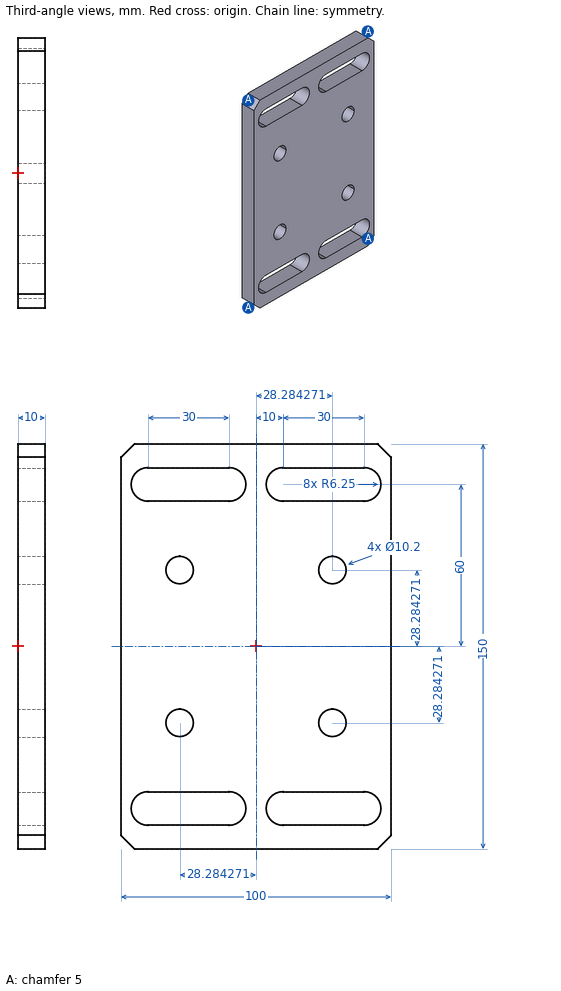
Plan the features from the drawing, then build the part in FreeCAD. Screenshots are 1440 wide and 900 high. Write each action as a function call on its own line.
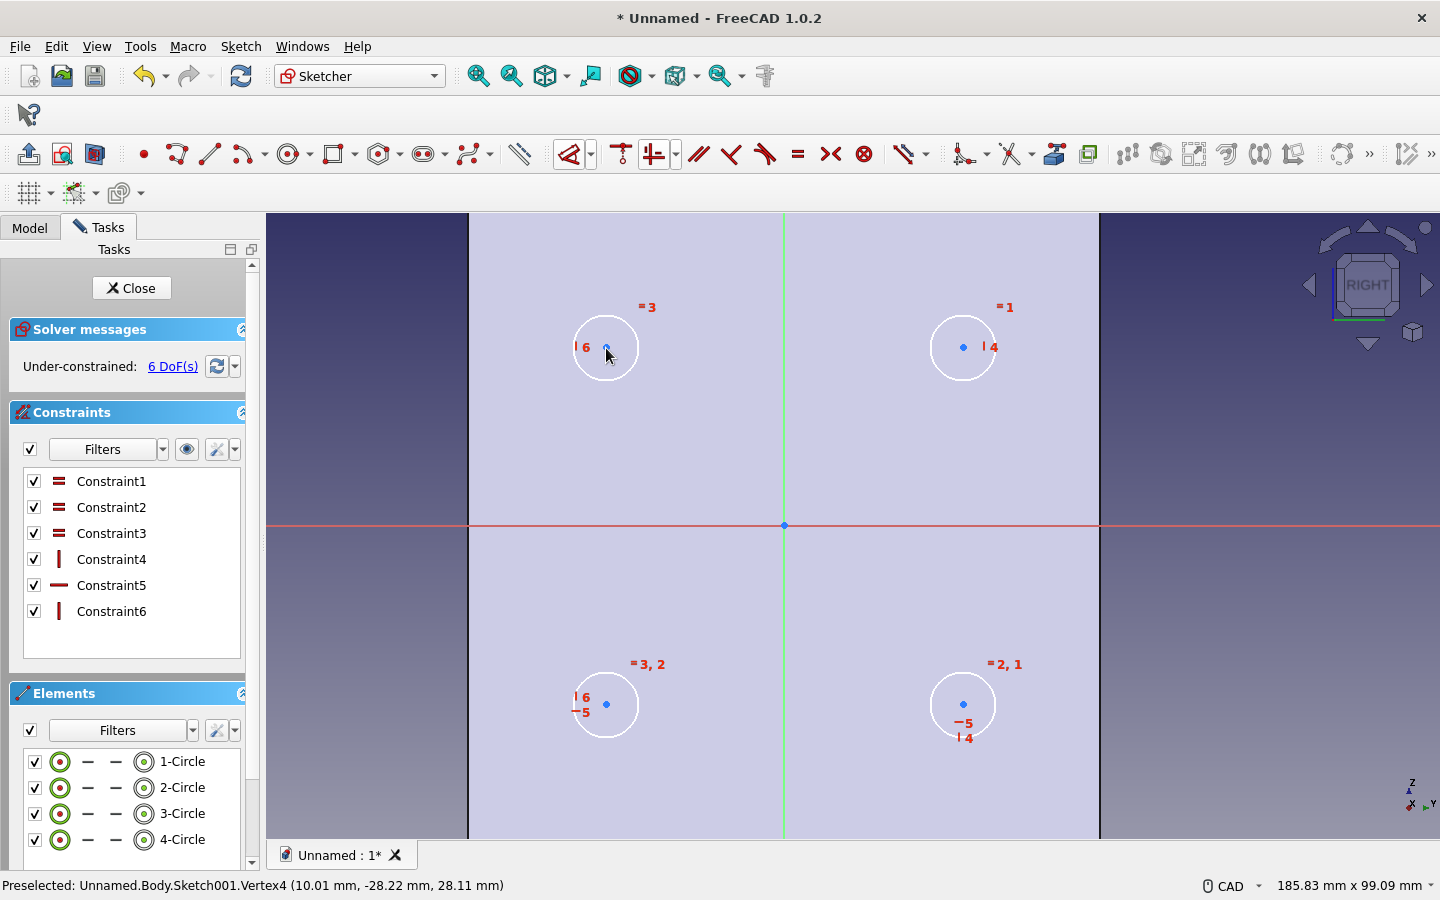
click(963, 348)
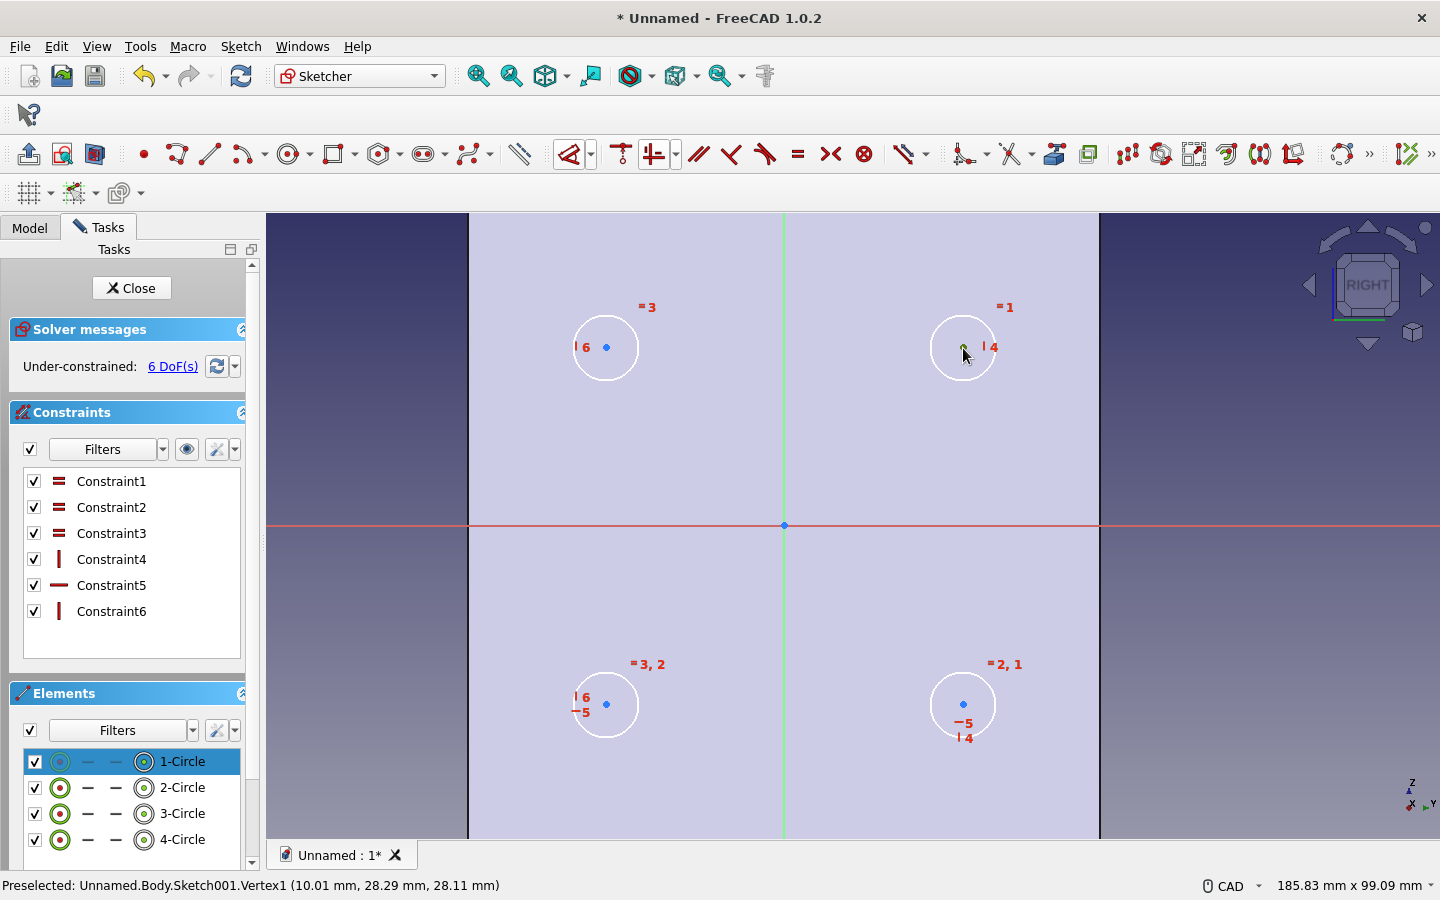
click(606, 348)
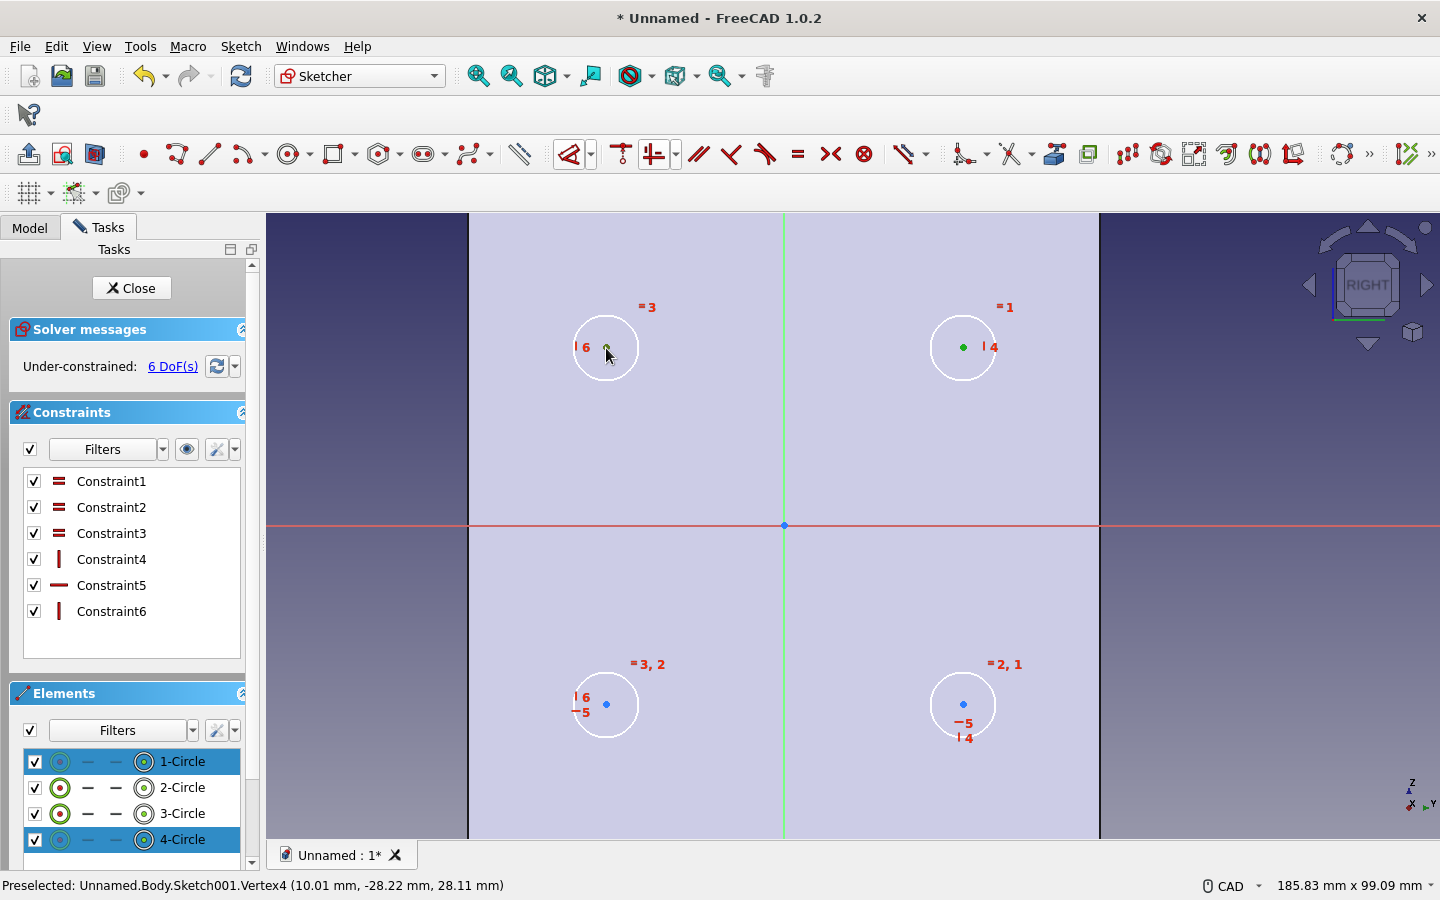
click(676, 154)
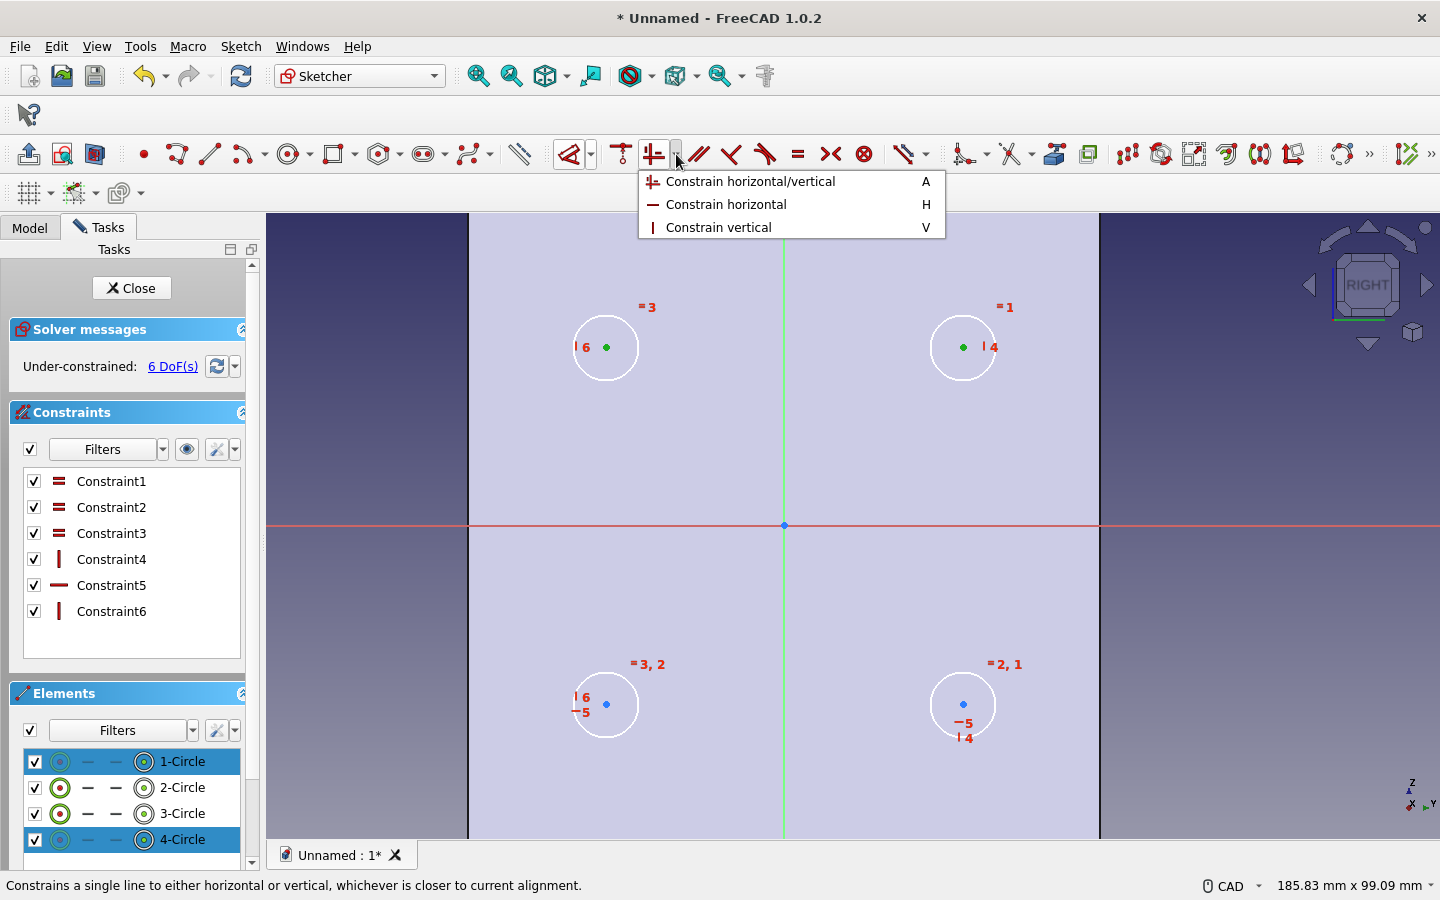
click(792, 204)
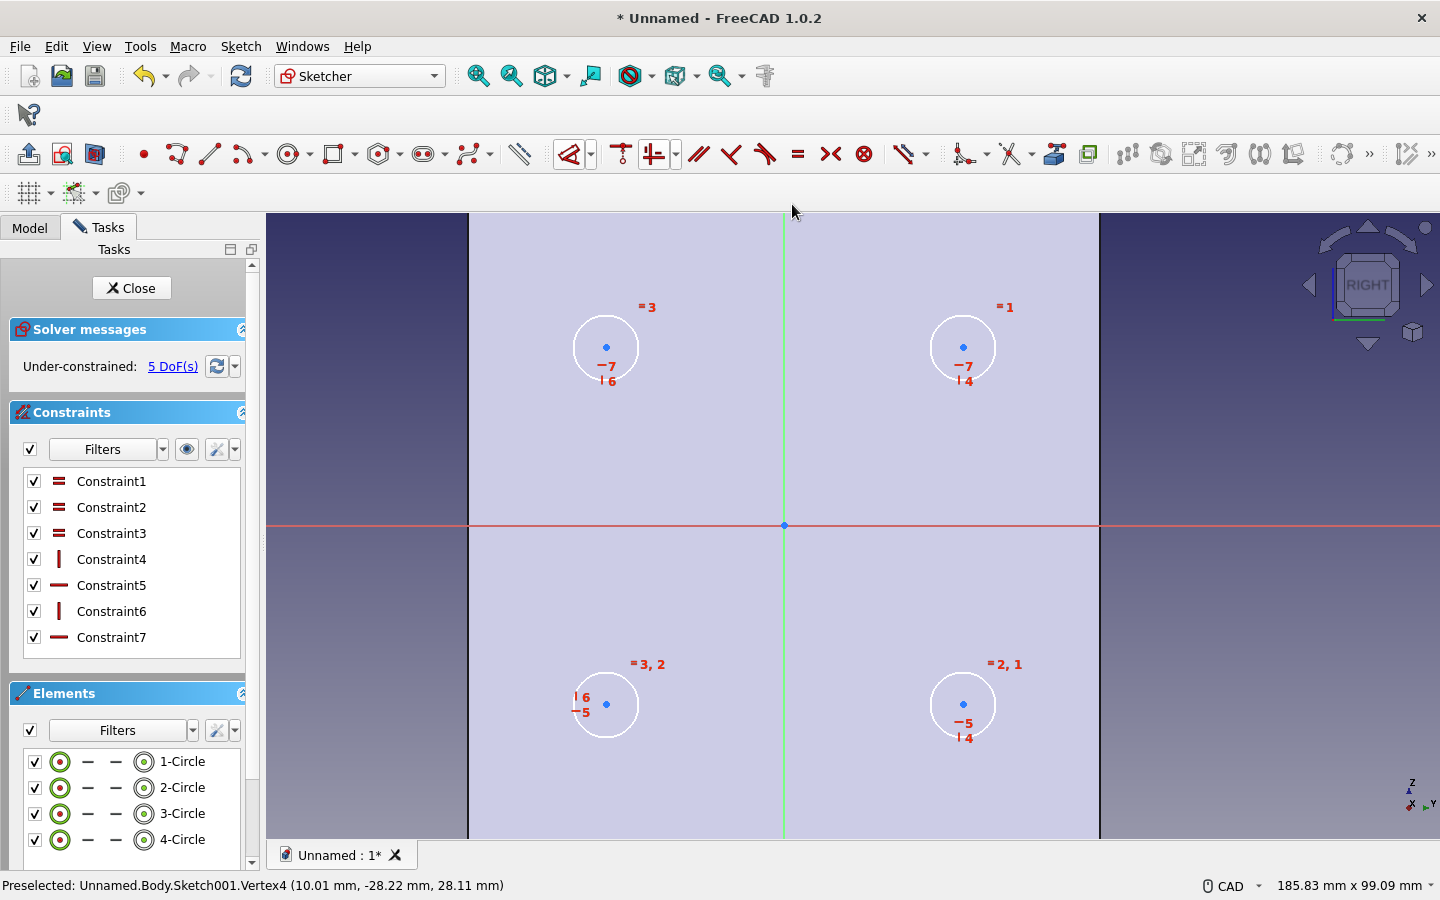
click(568, 154)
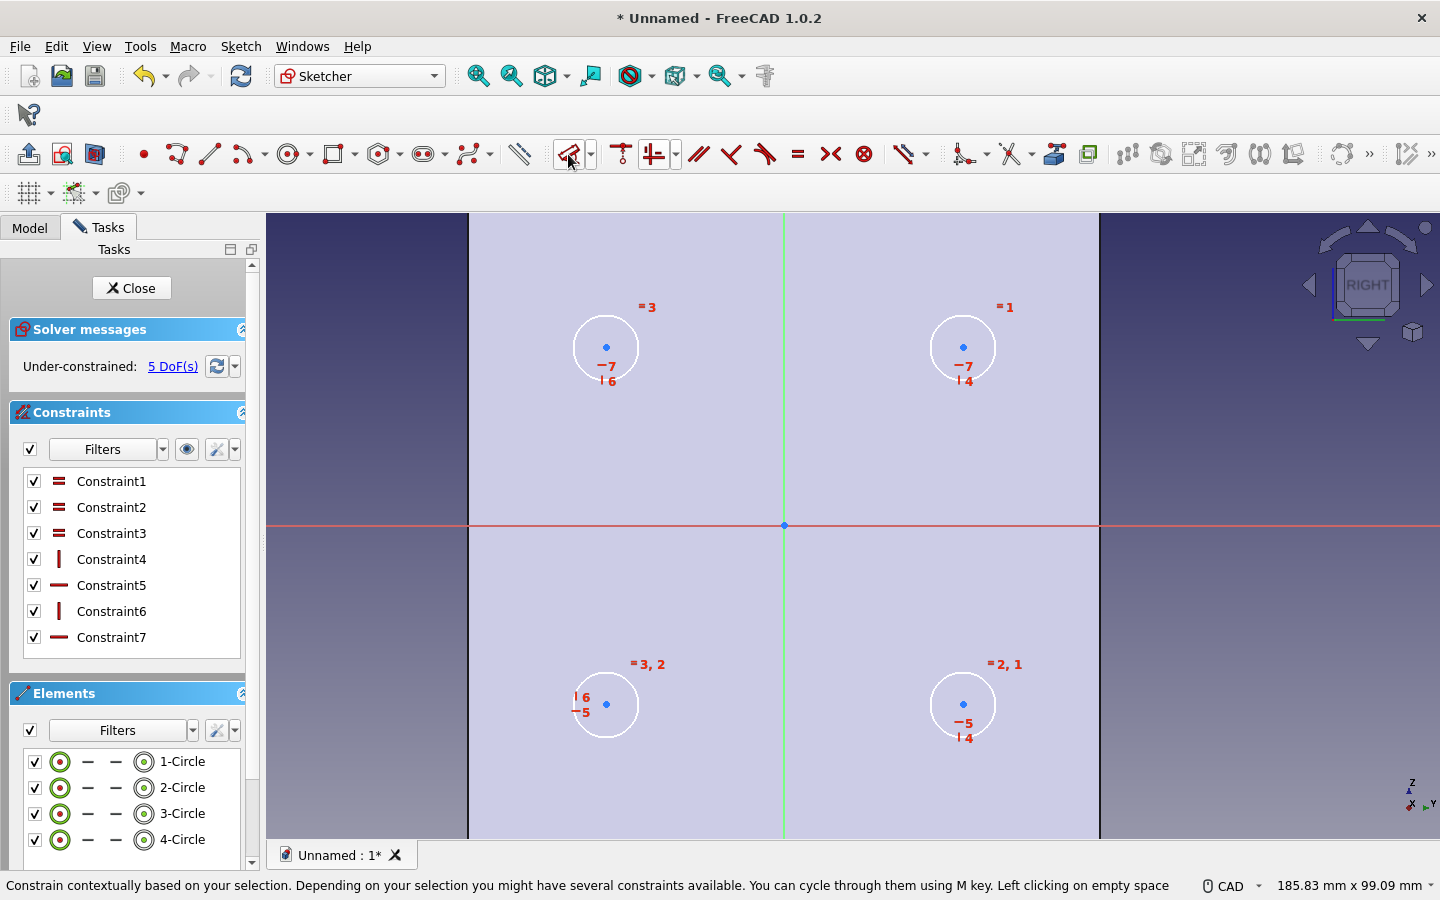
click(986, 325)
click(1009, 302)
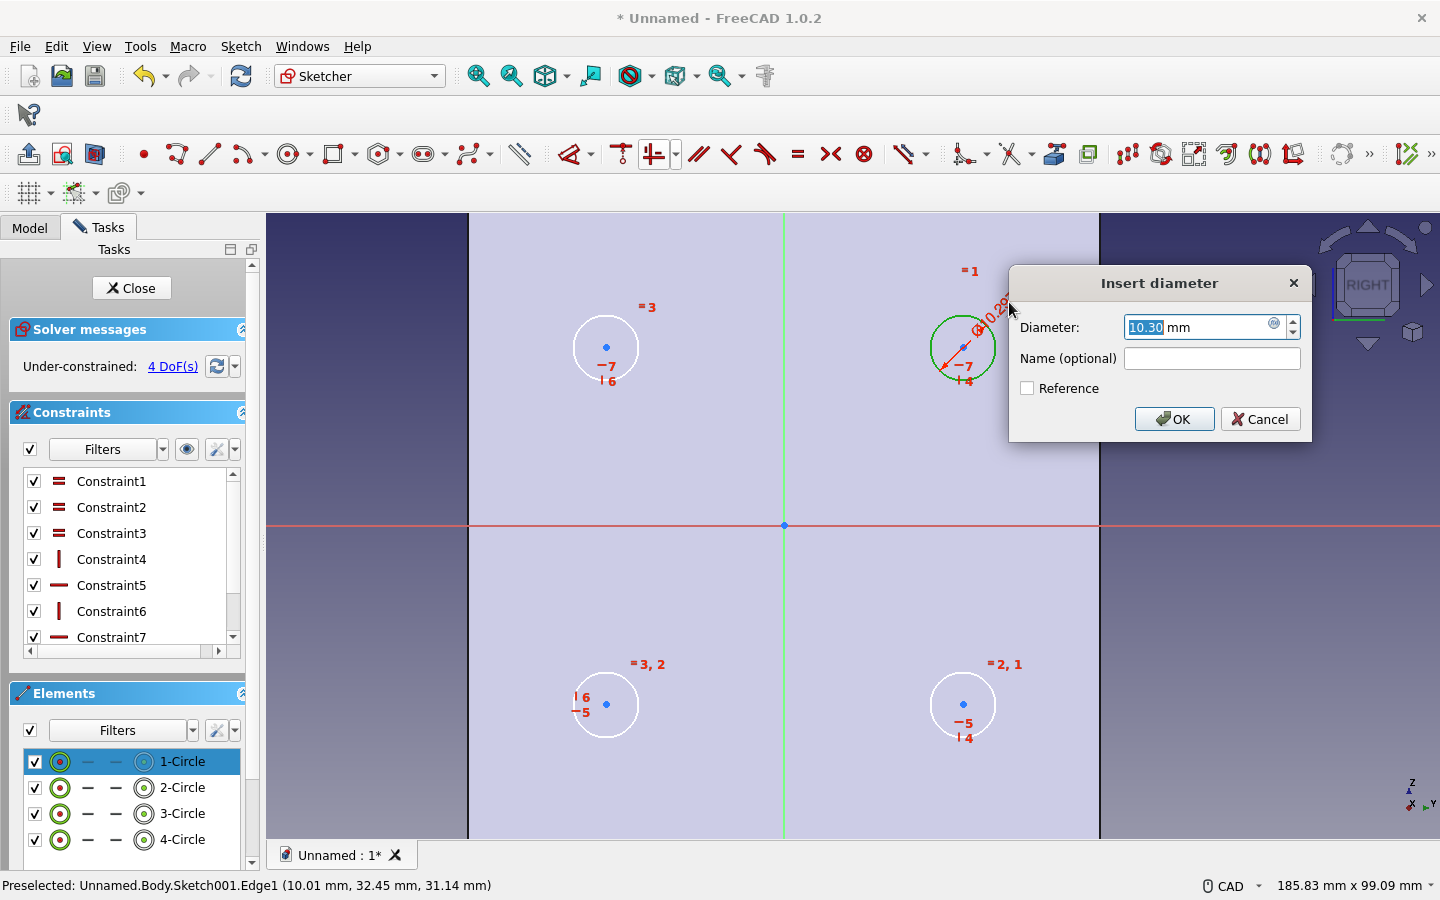
text(10.2)
key(Return)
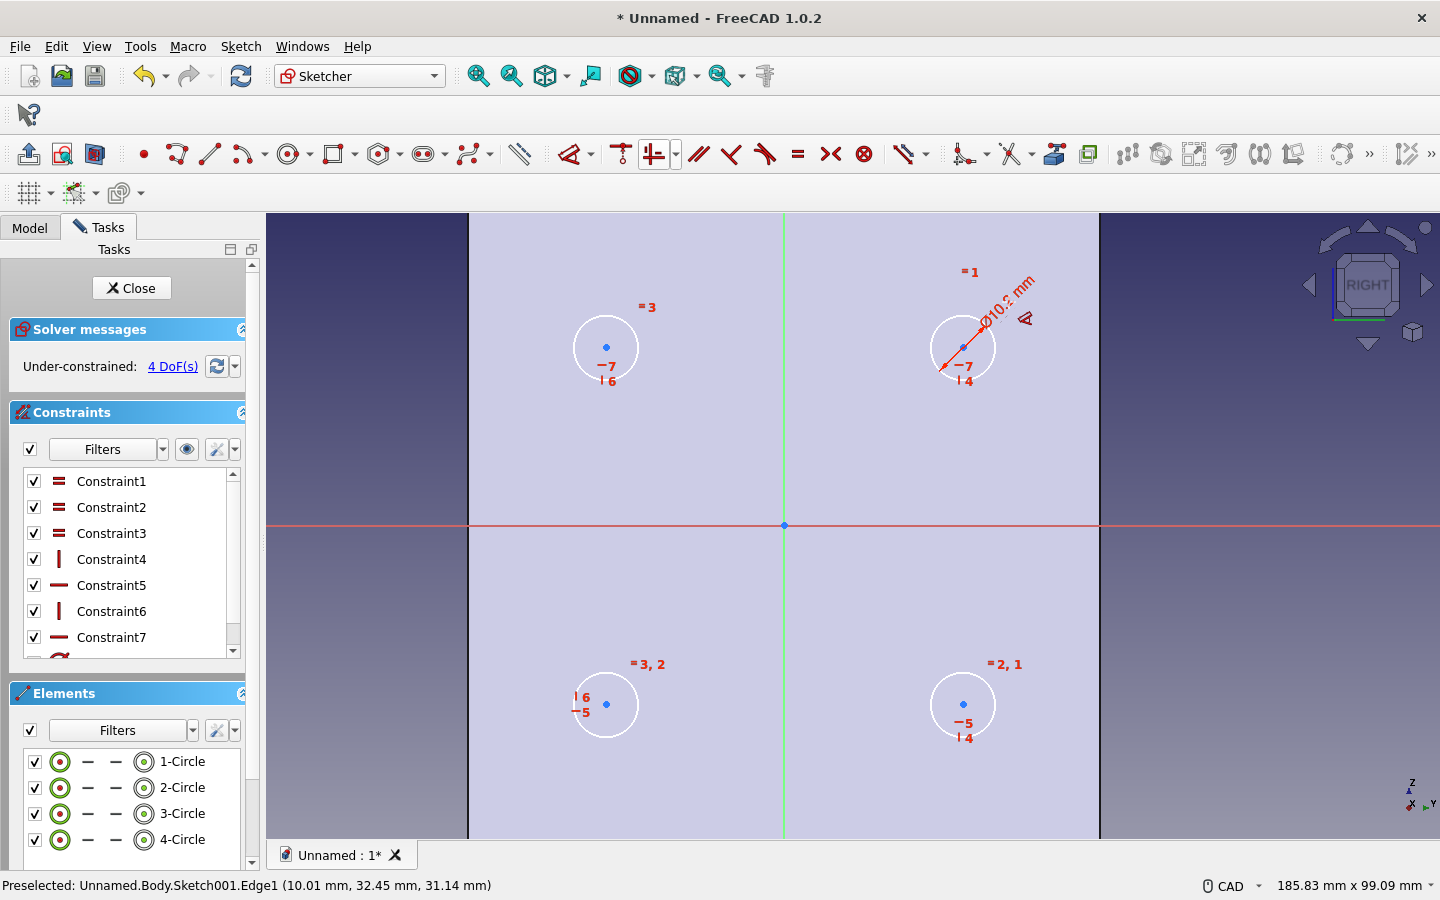
click(963, 348)
click(874, 314)